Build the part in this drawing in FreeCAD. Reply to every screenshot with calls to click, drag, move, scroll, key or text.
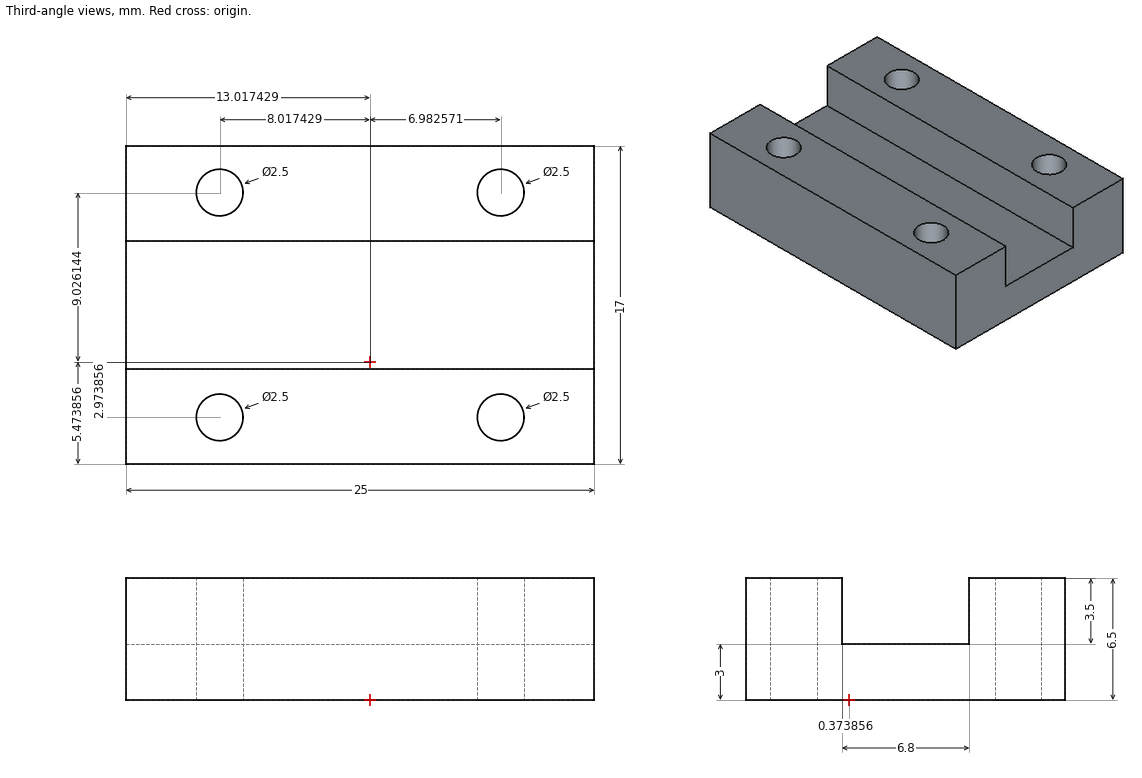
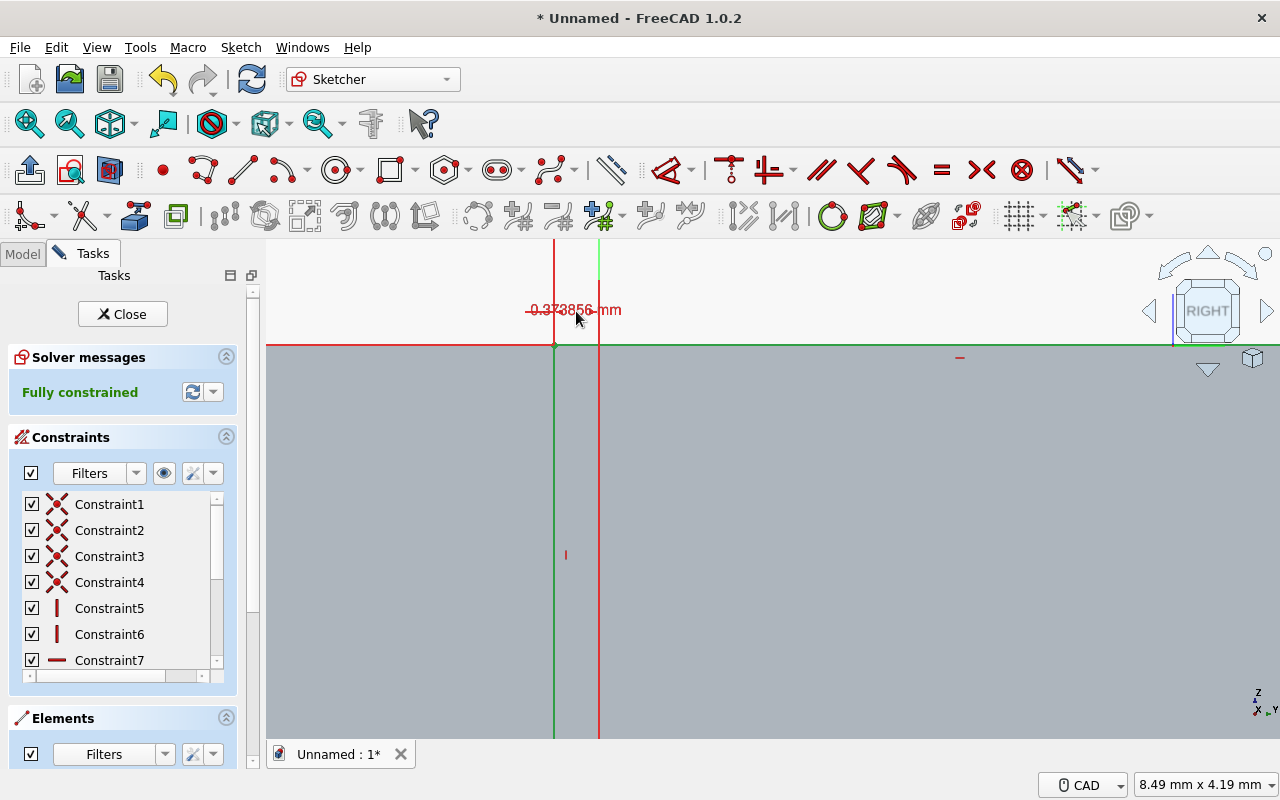
click(123, 314)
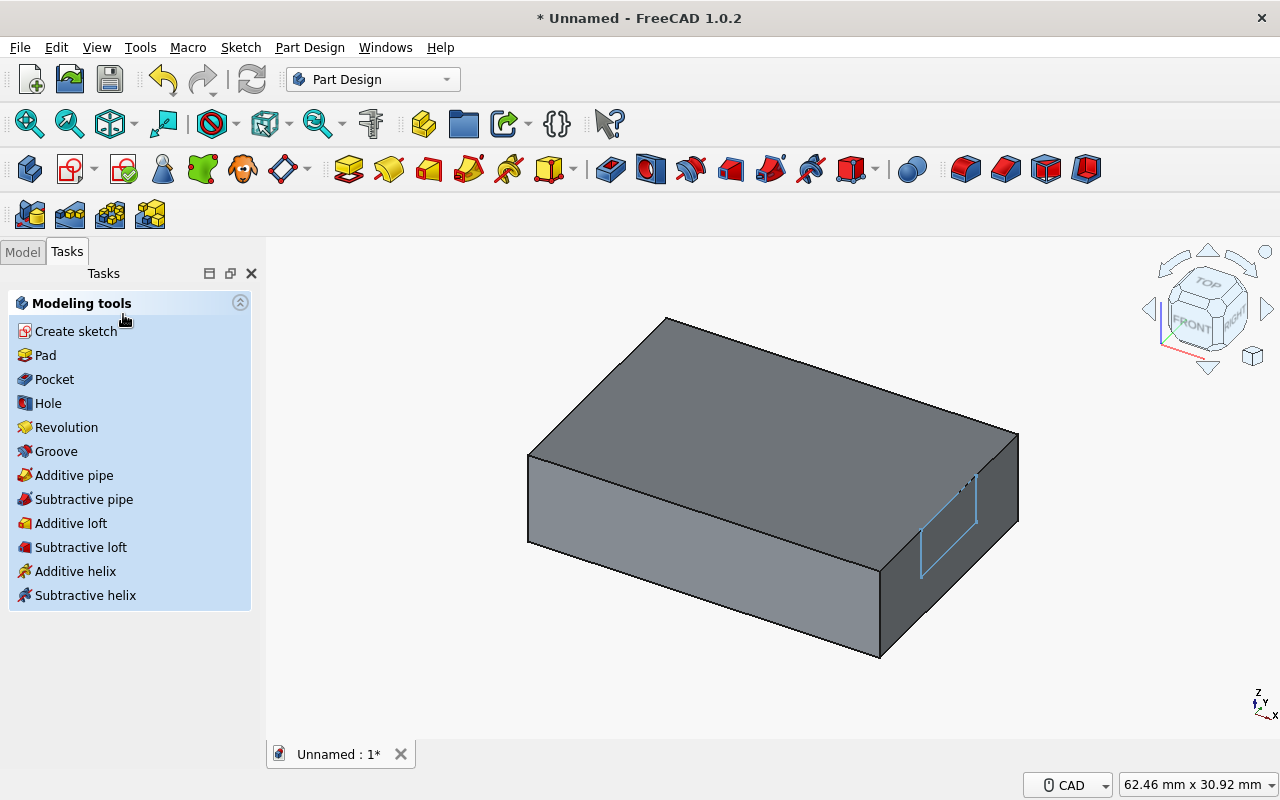
click(612, 170)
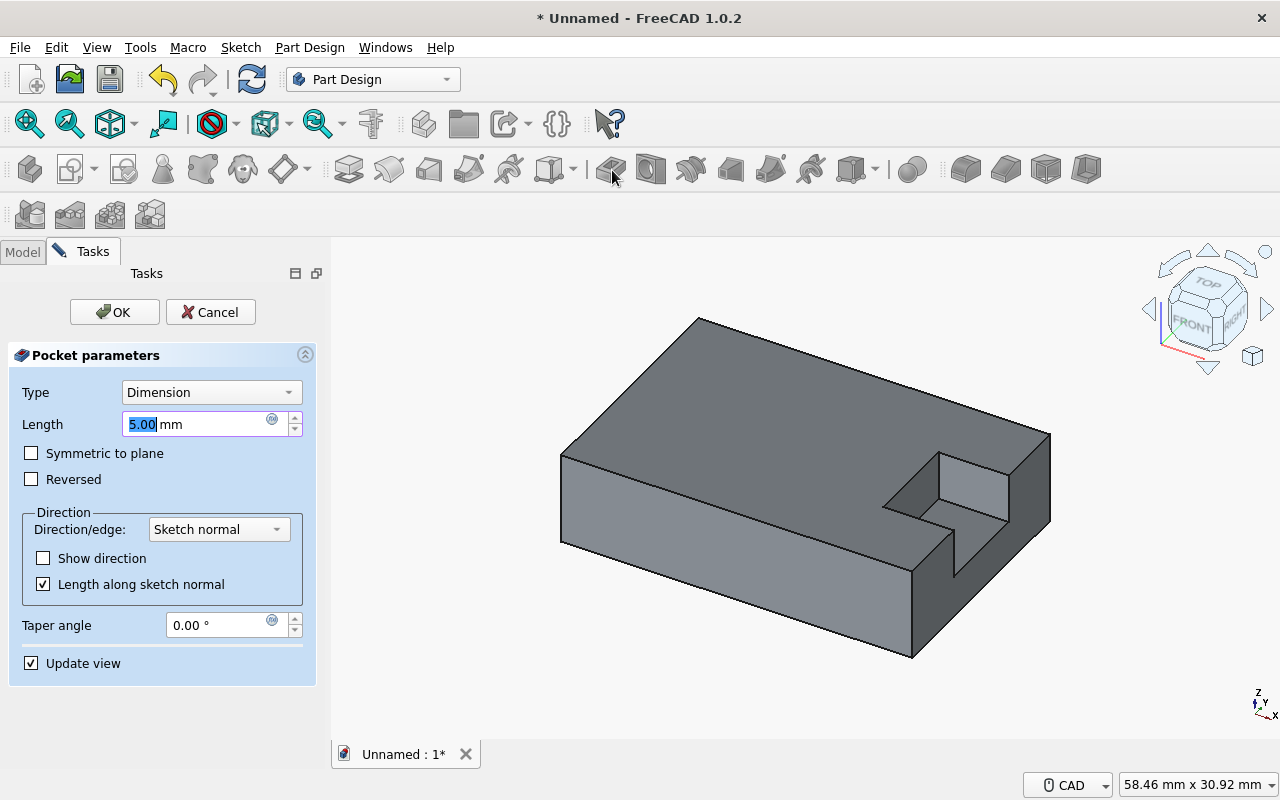
click(212, 392)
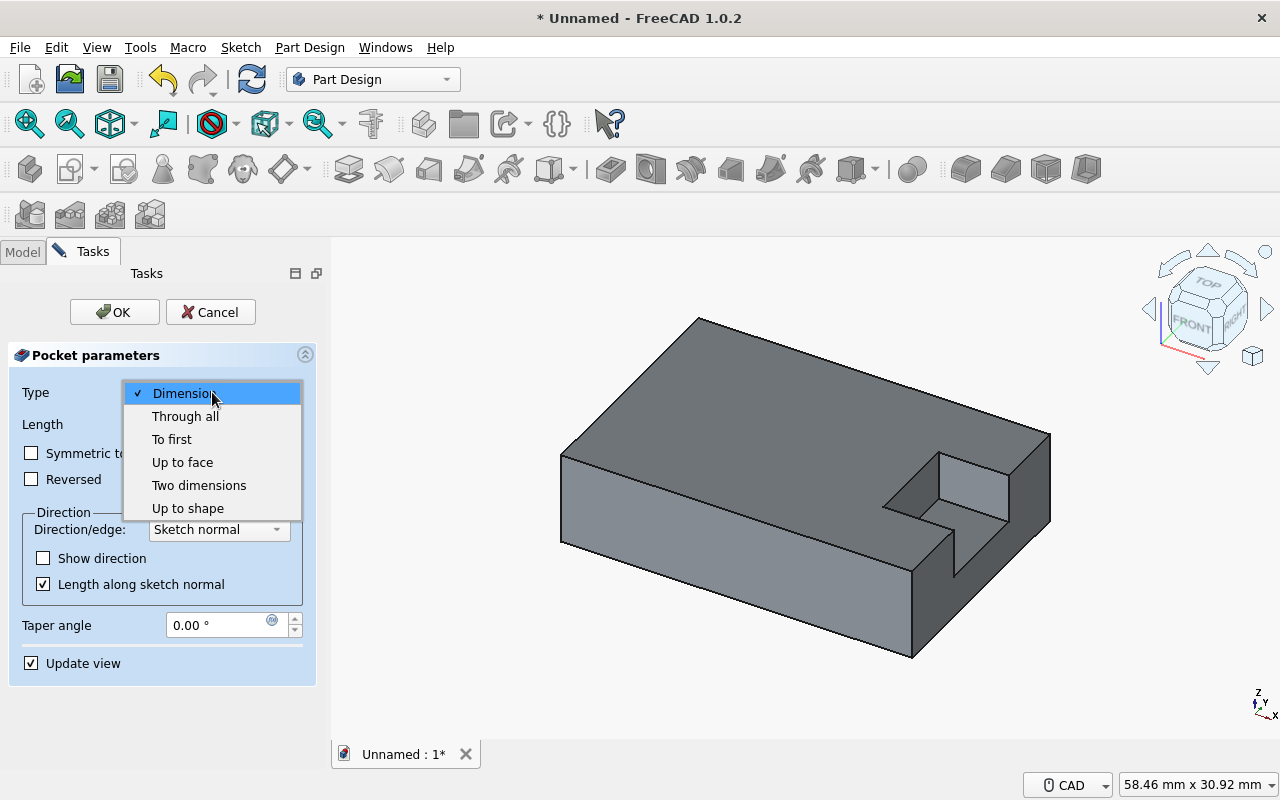
click(212, 440)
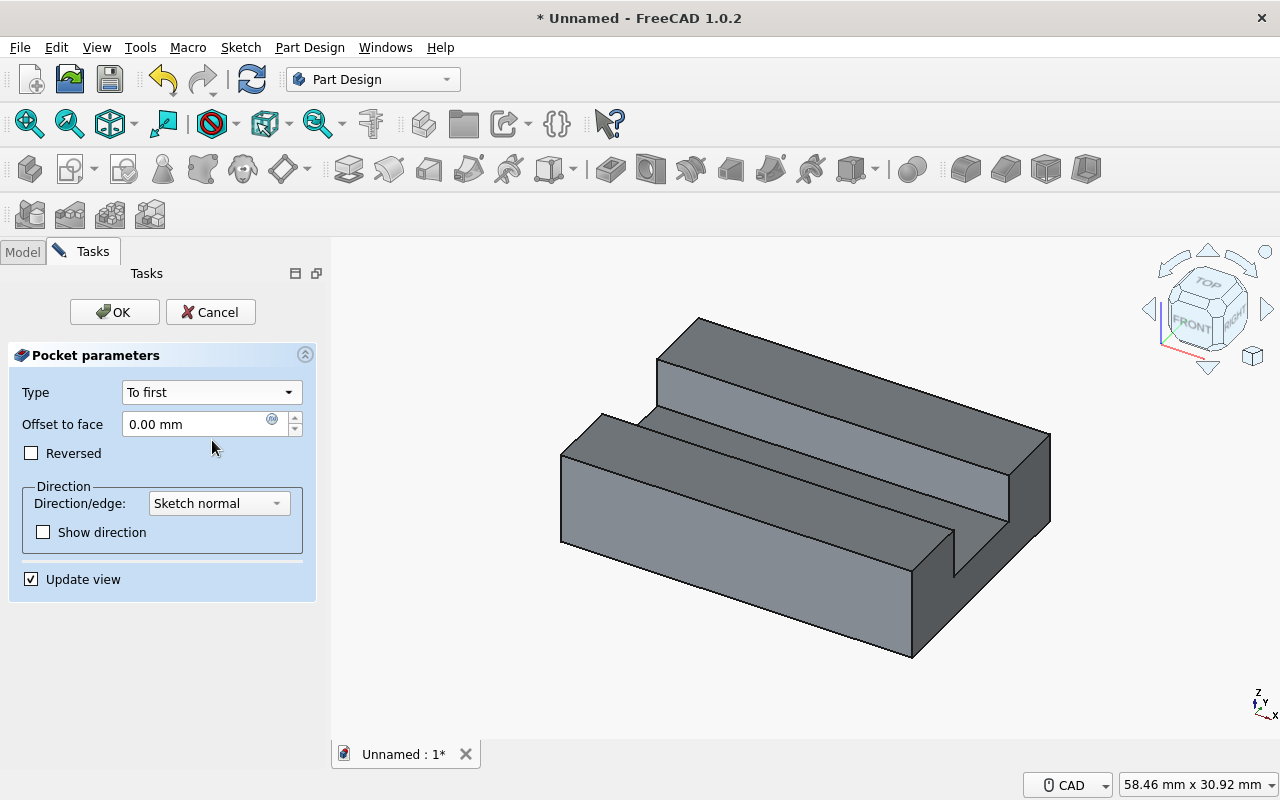
click(115, 312)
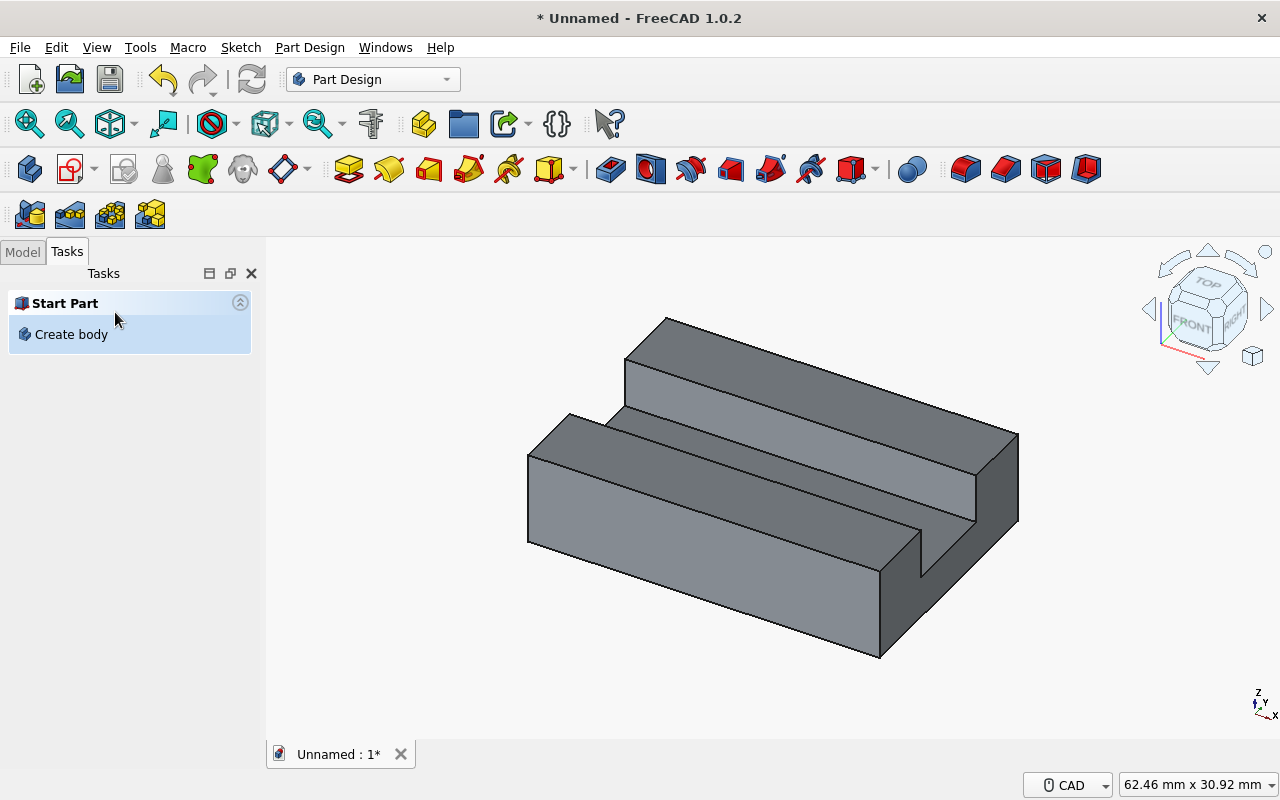
click(922, 429)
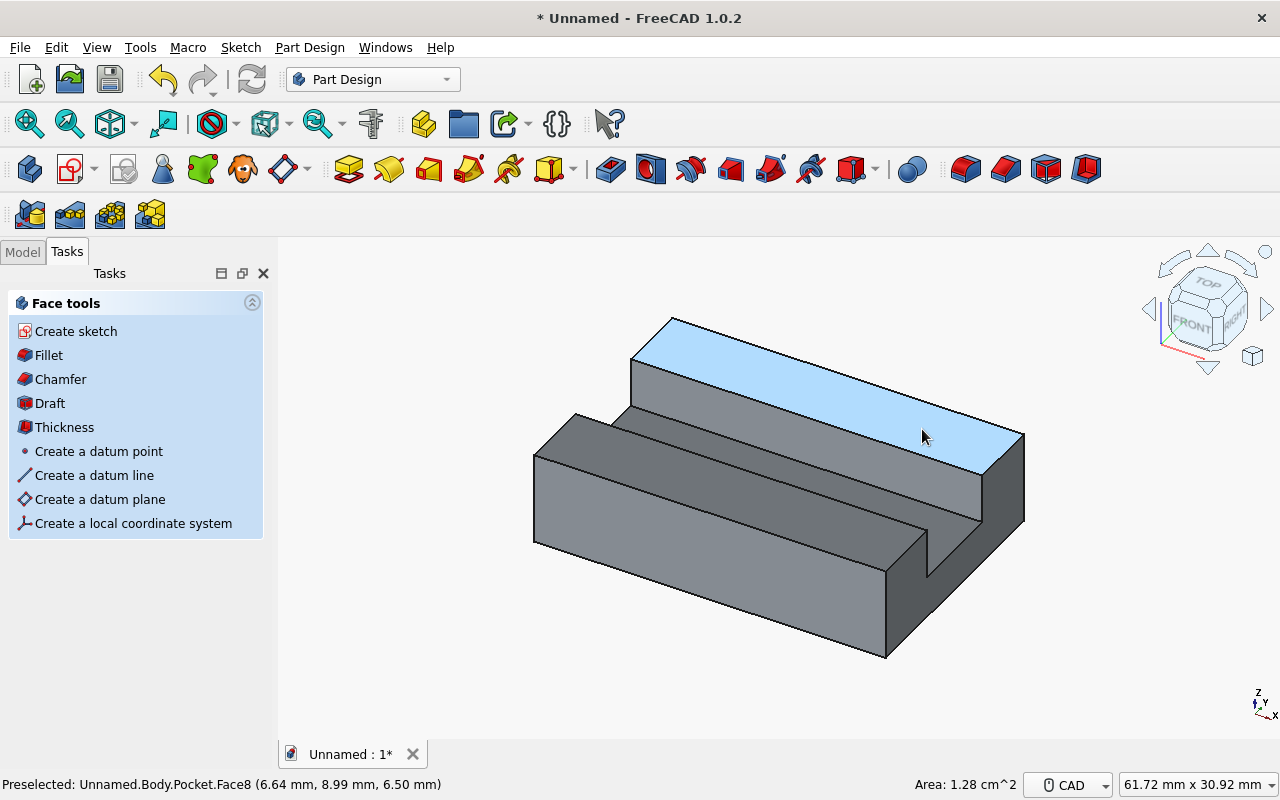
click(70, 170)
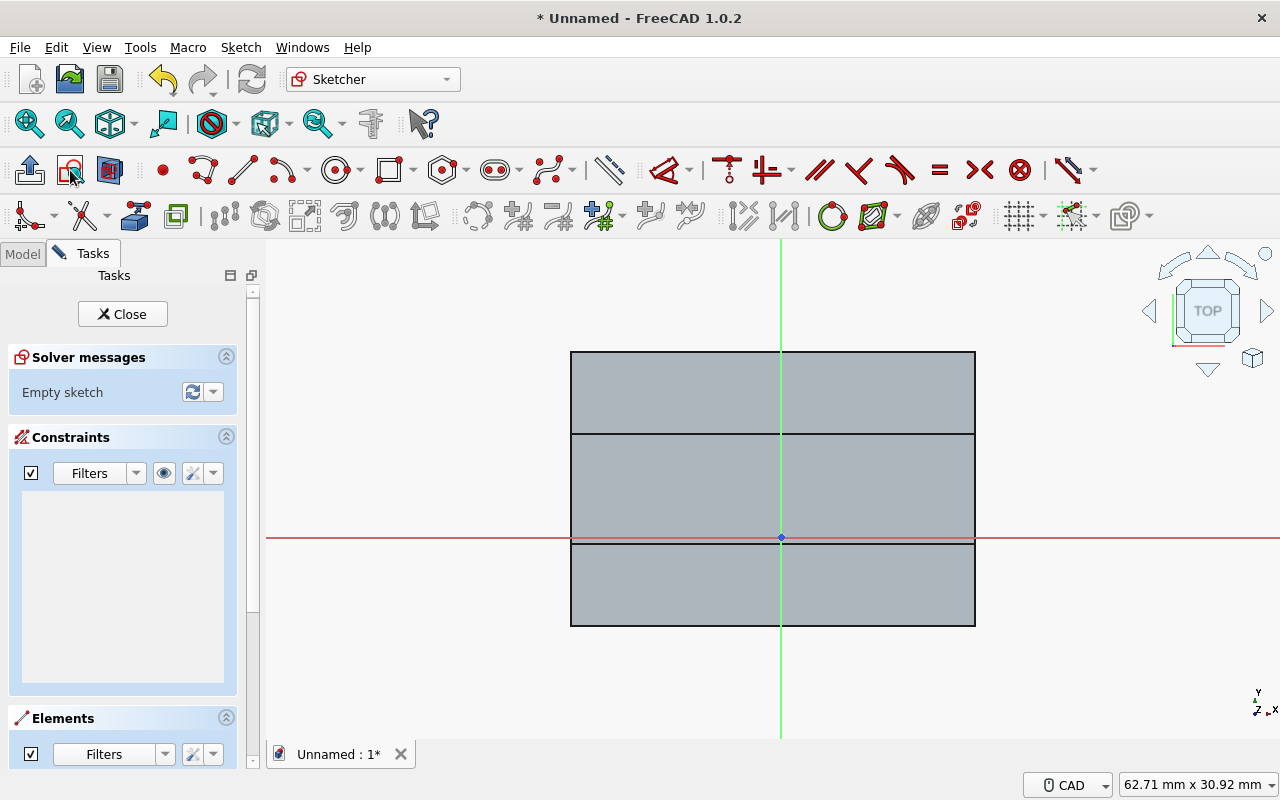
scroll(643, 377, up, 10)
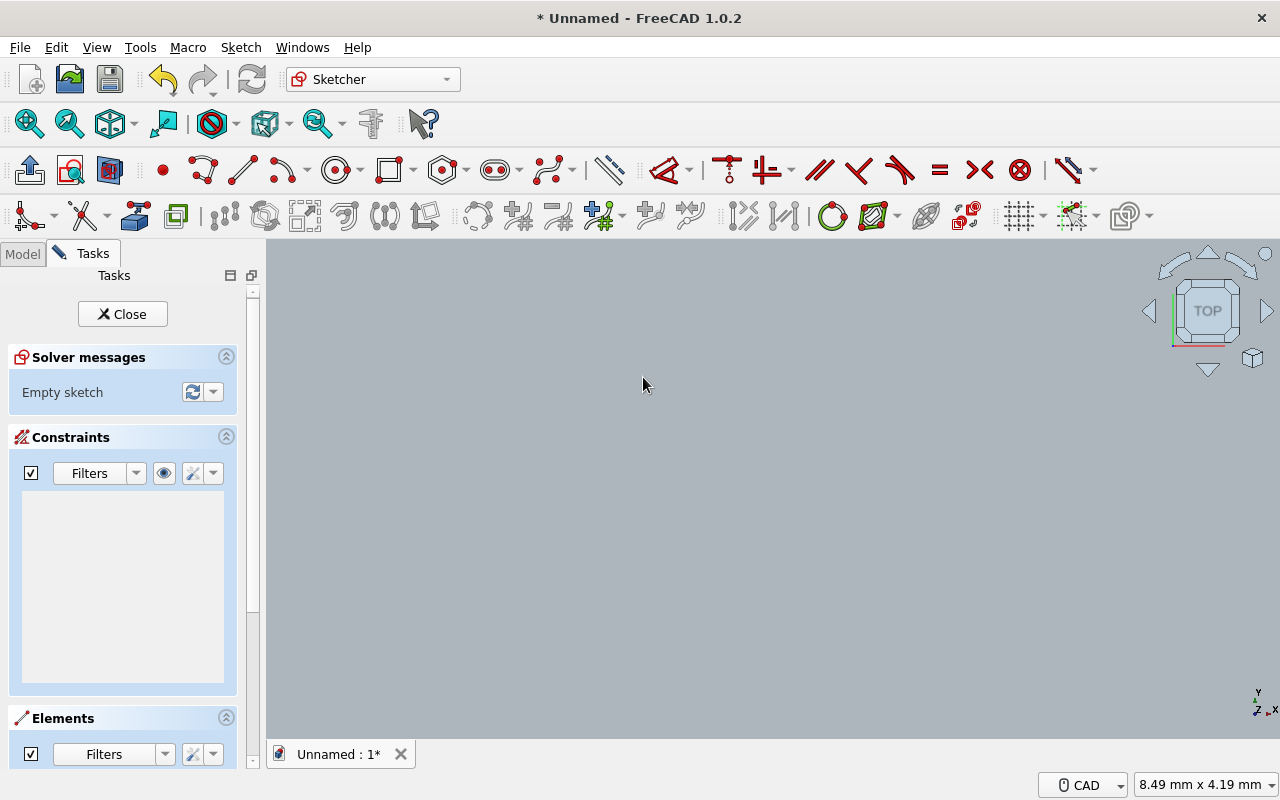
click(336, 170)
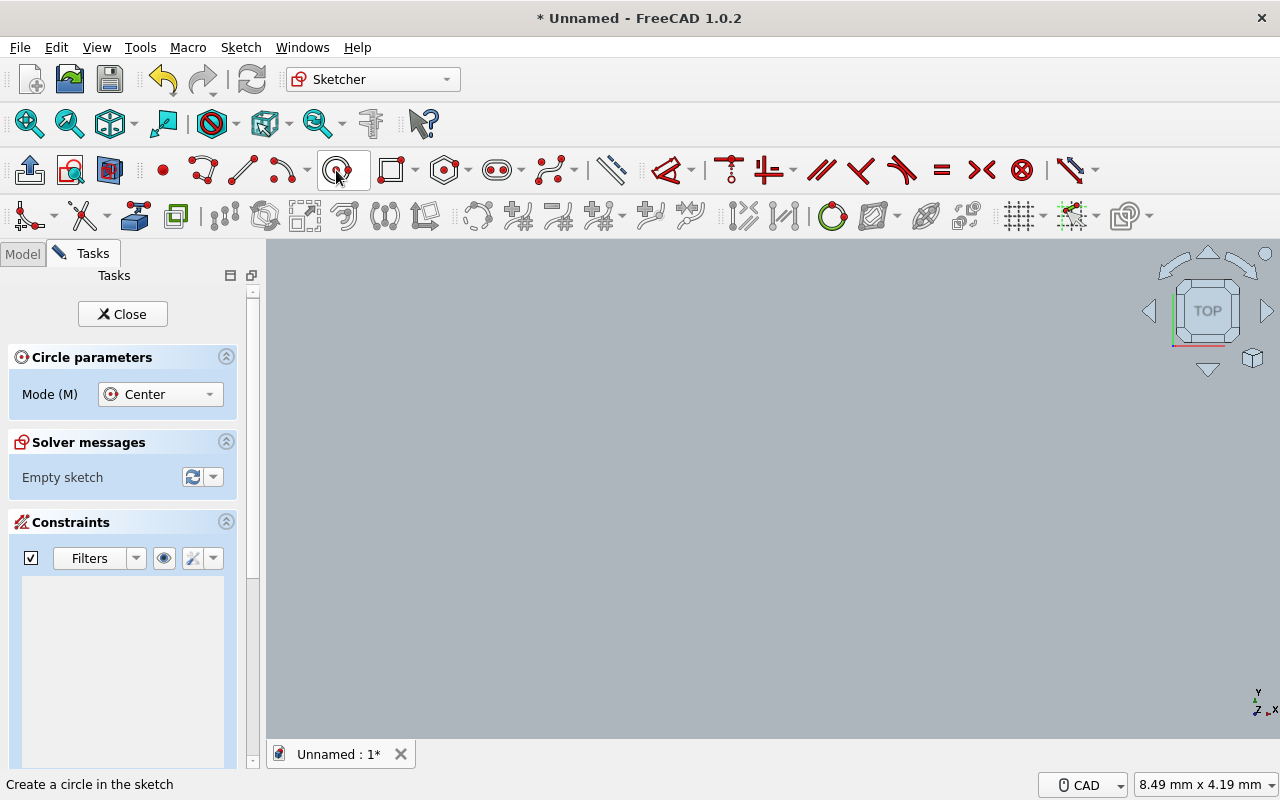
click(705, 486)
move(811, 380)